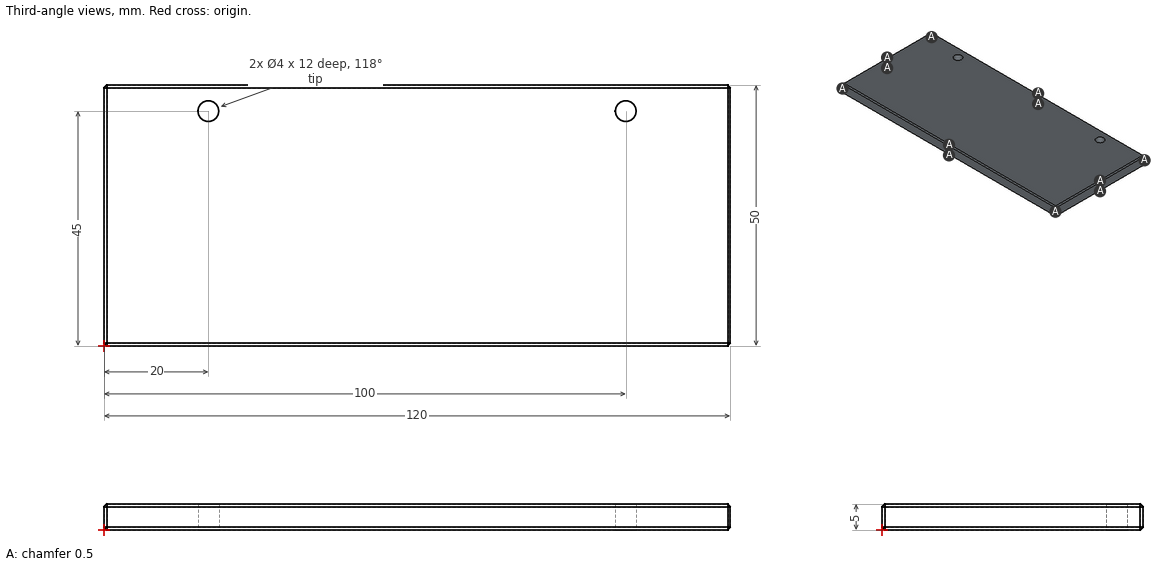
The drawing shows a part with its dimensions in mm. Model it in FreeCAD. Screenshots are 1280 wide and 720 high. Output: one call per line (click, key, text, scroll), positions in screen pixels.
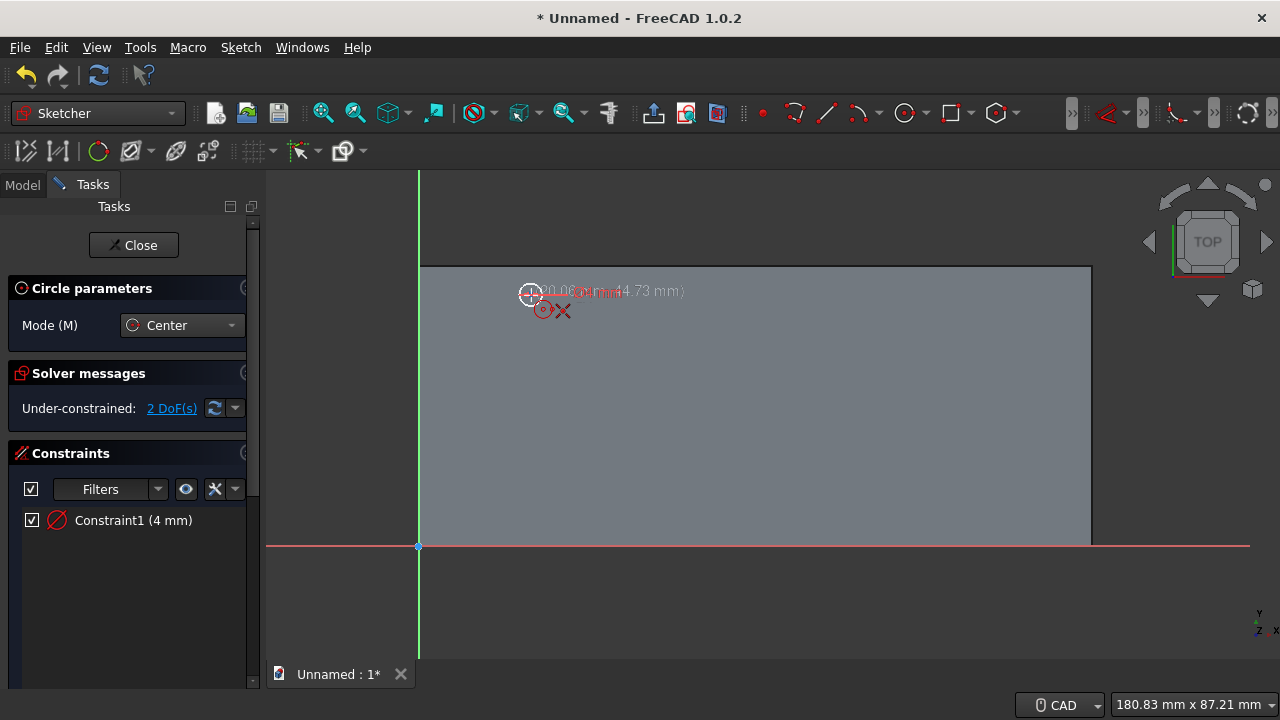
scroll(979, 294, up, 4)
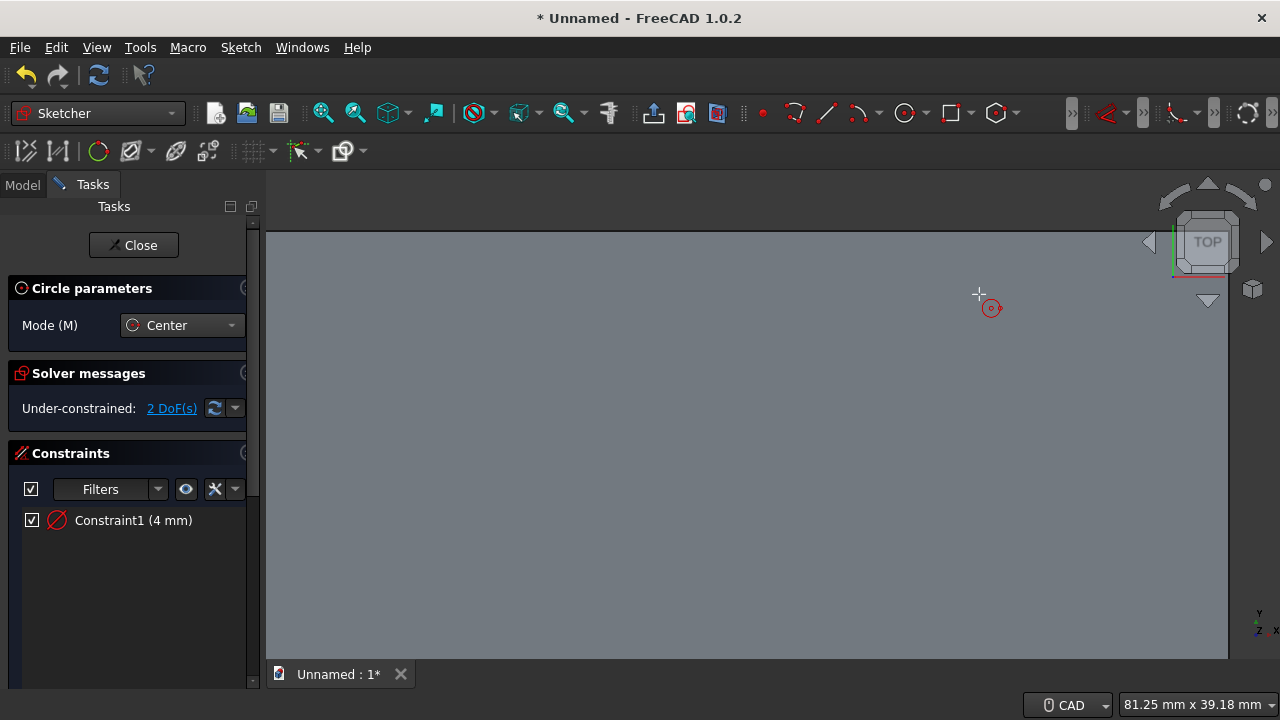
click(979, 294)
move(997, 276)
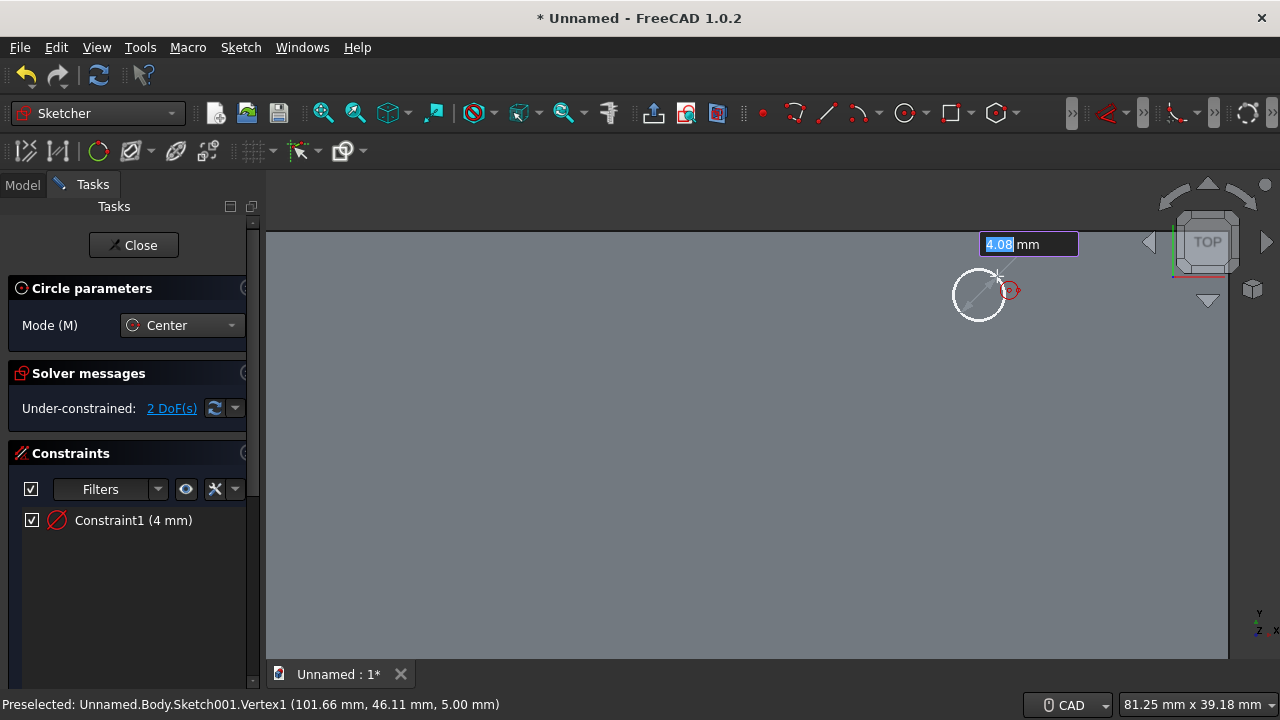
text(4)
key(Return)
key(Escape)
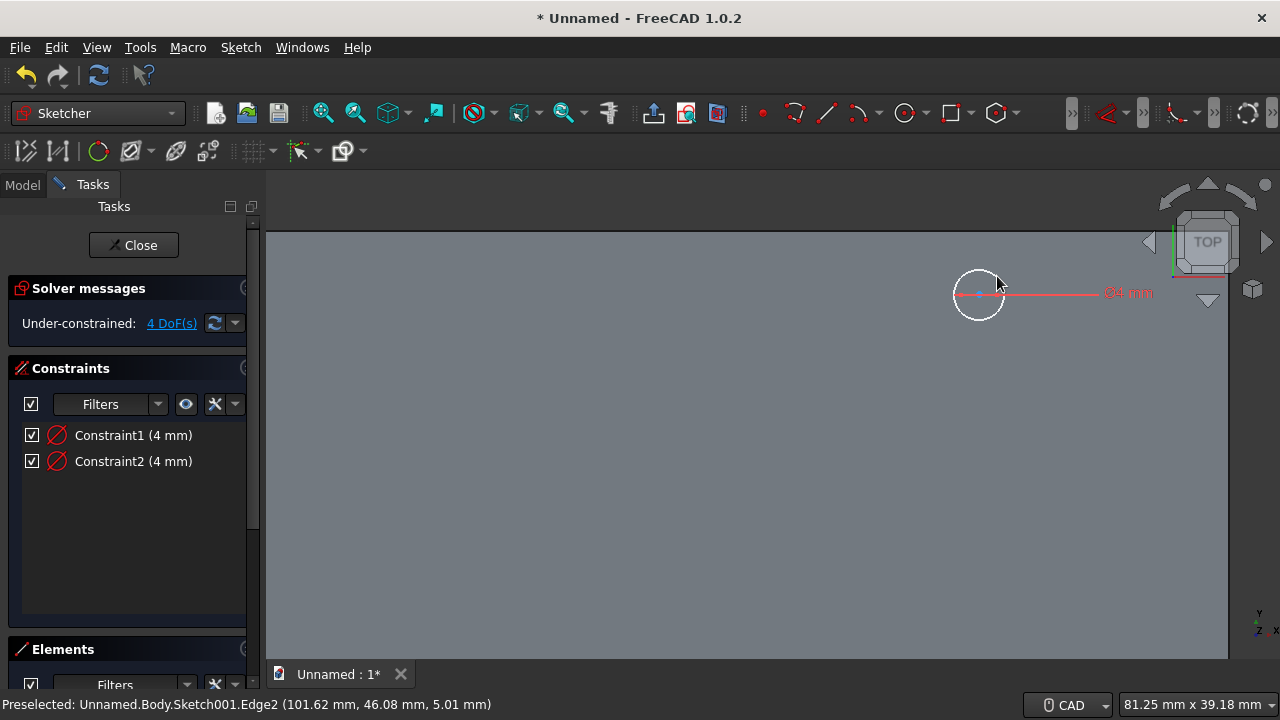
key(d)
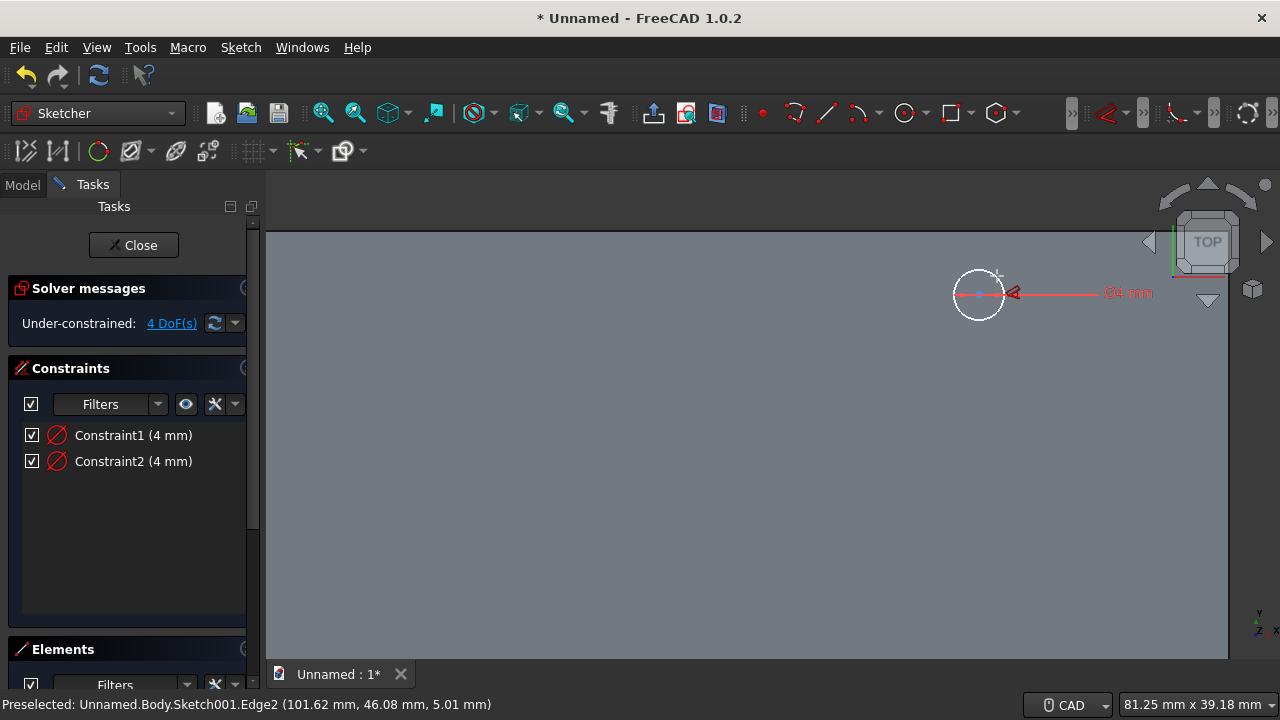
scroll(979, 294, down, 4)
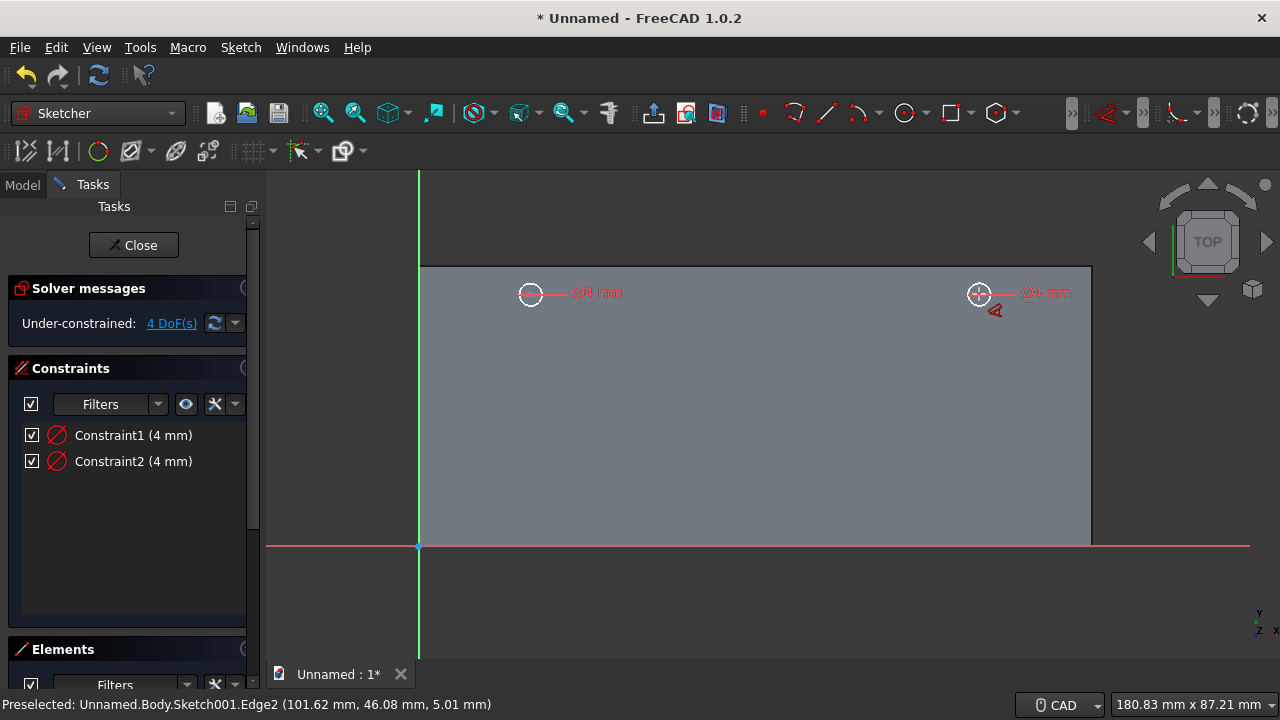
click(531, 295)
click(475, 580)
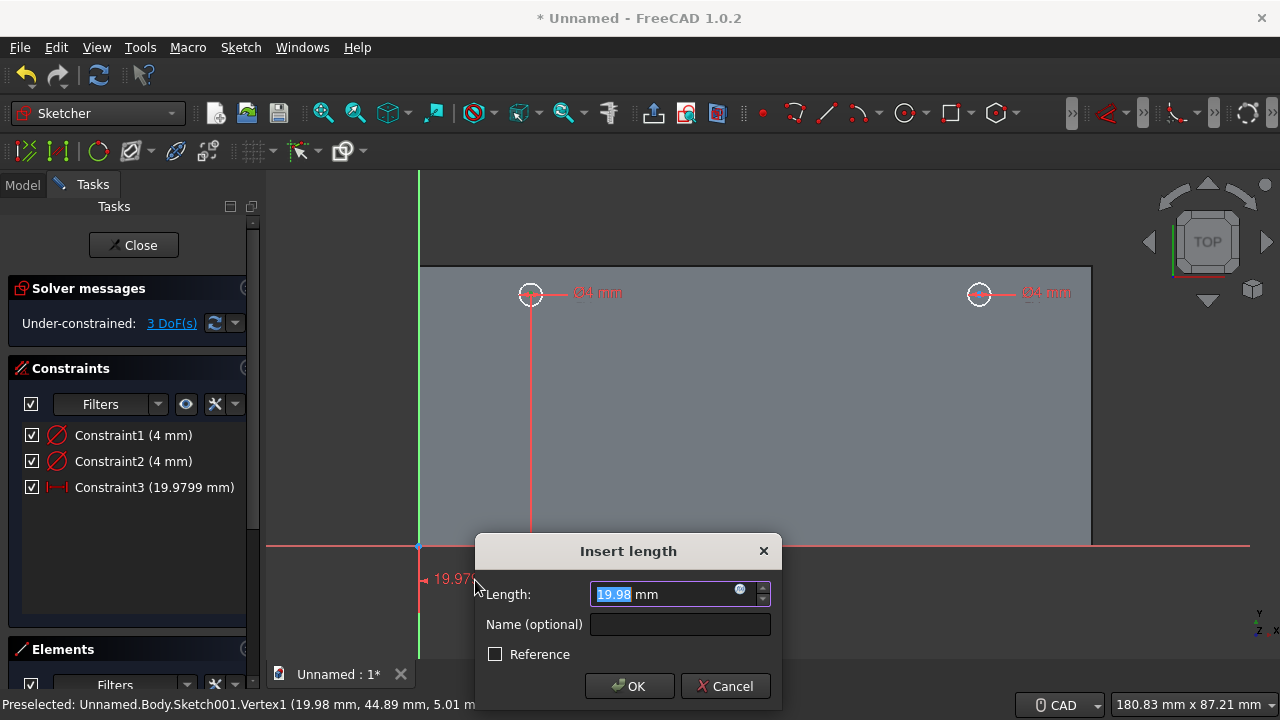
text(20)
key(Return)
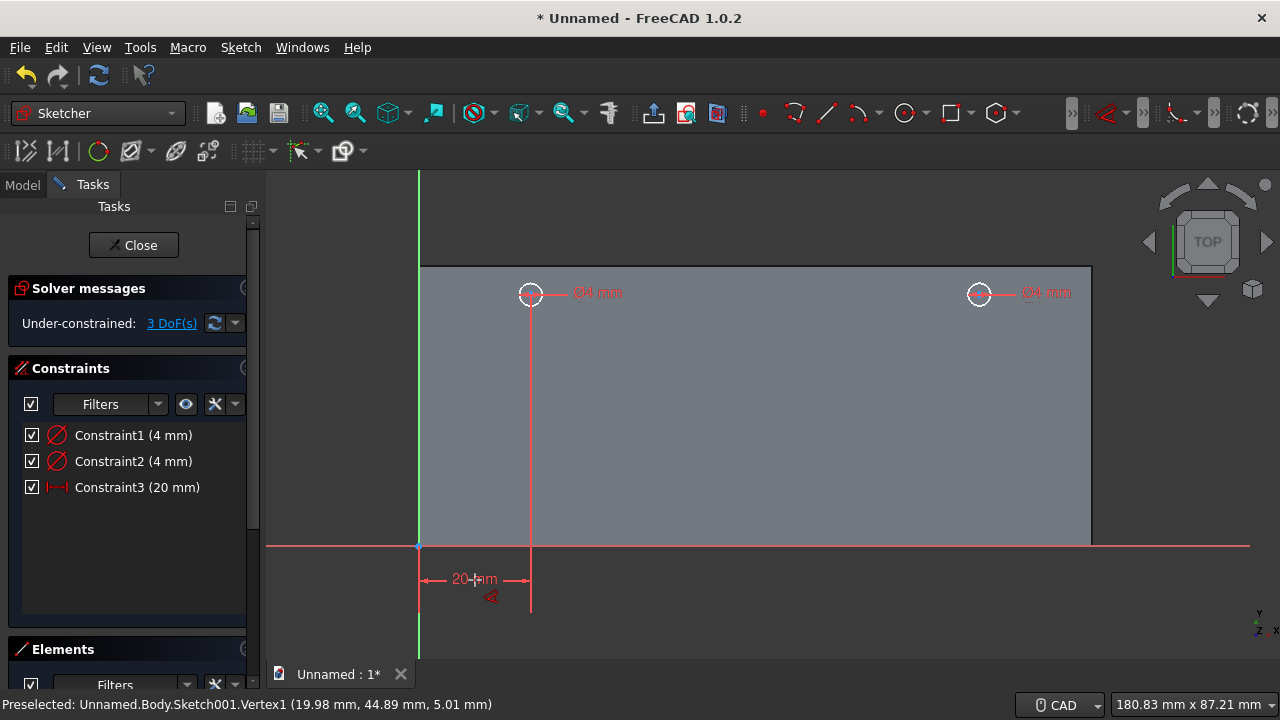
click(531, 295)
click(385, 421)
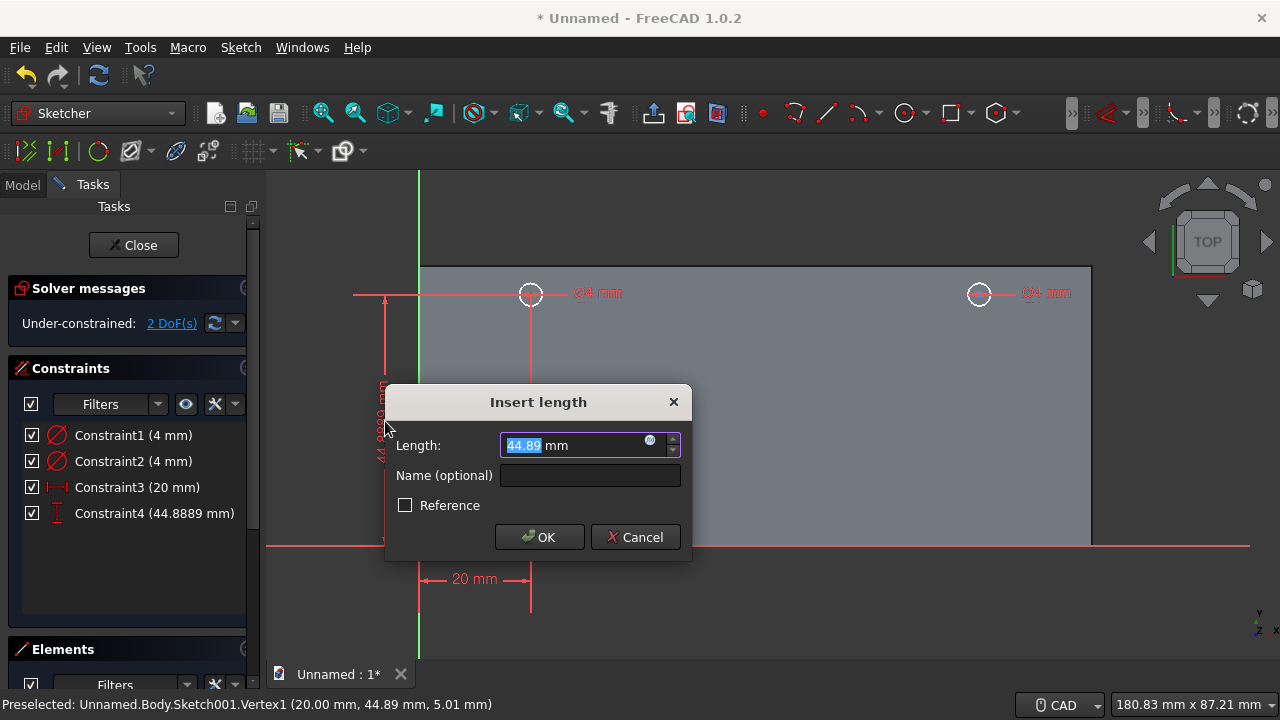
text(45)
key(Return)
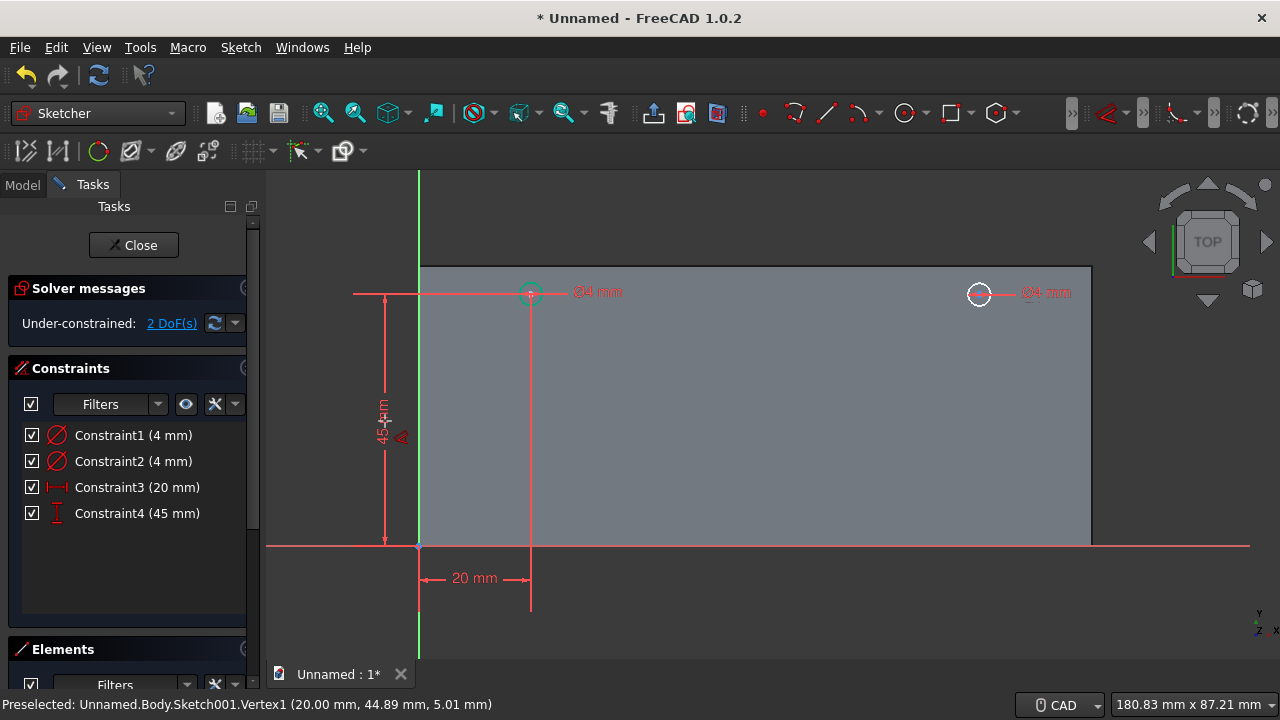
click(979, 295)
click(385, 363)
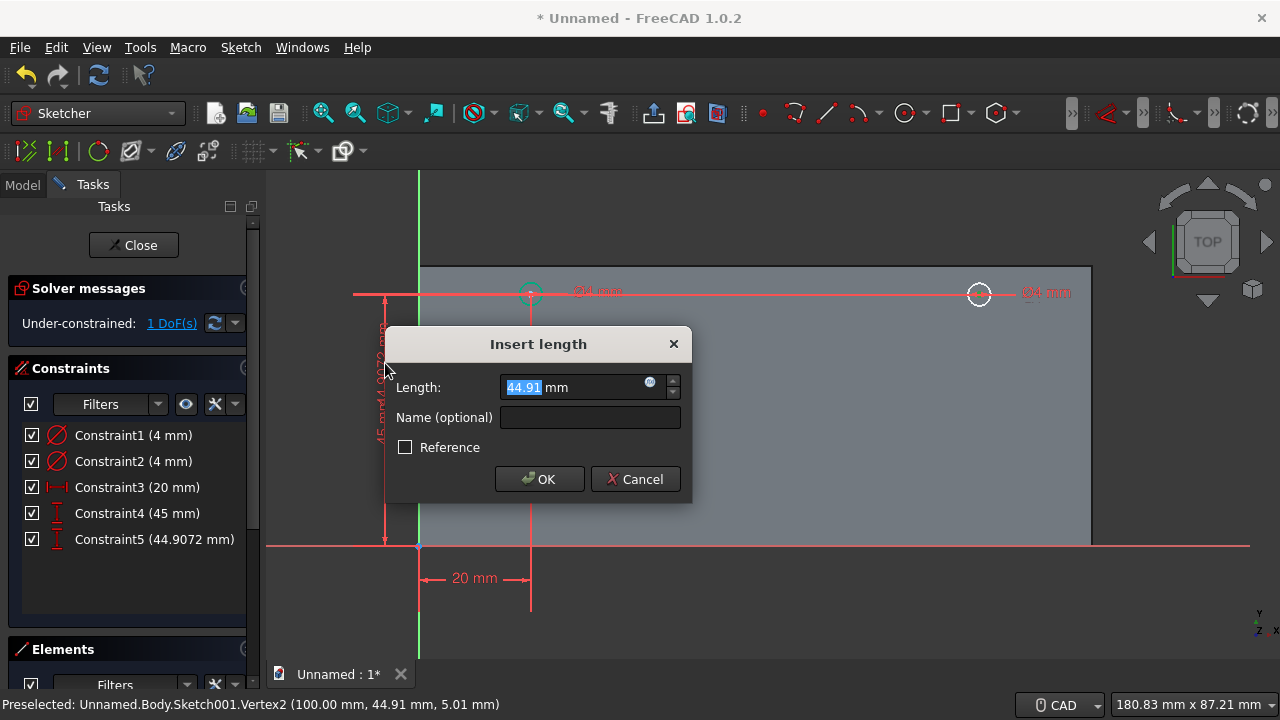
text(45)
key(Return)